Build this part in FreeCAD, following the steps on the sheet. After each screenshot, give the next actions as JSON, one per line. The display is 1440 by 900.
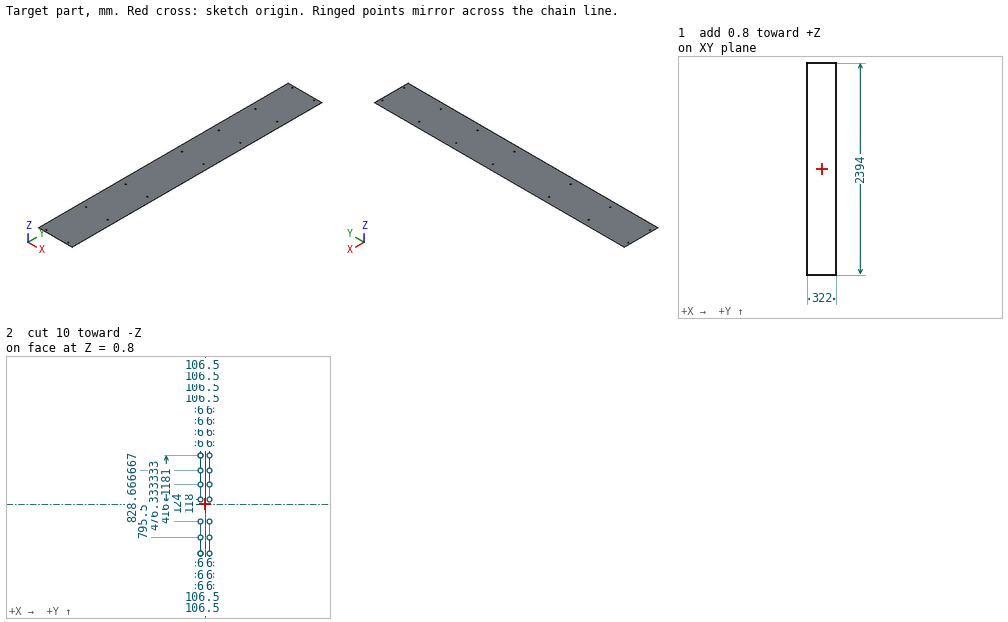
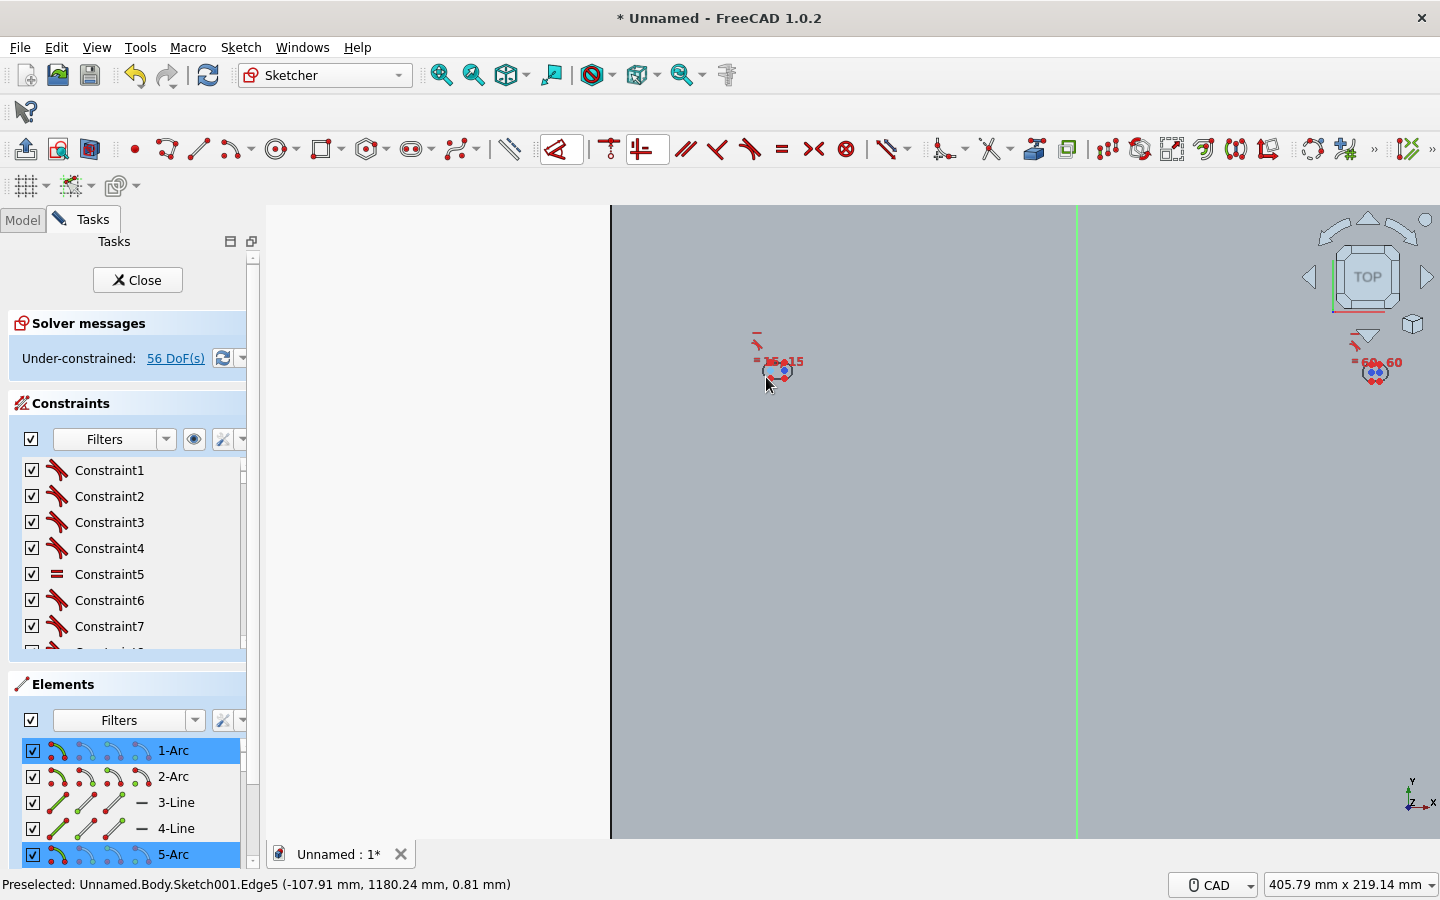
{"action": "left_click", "coordinate": [763, 371]}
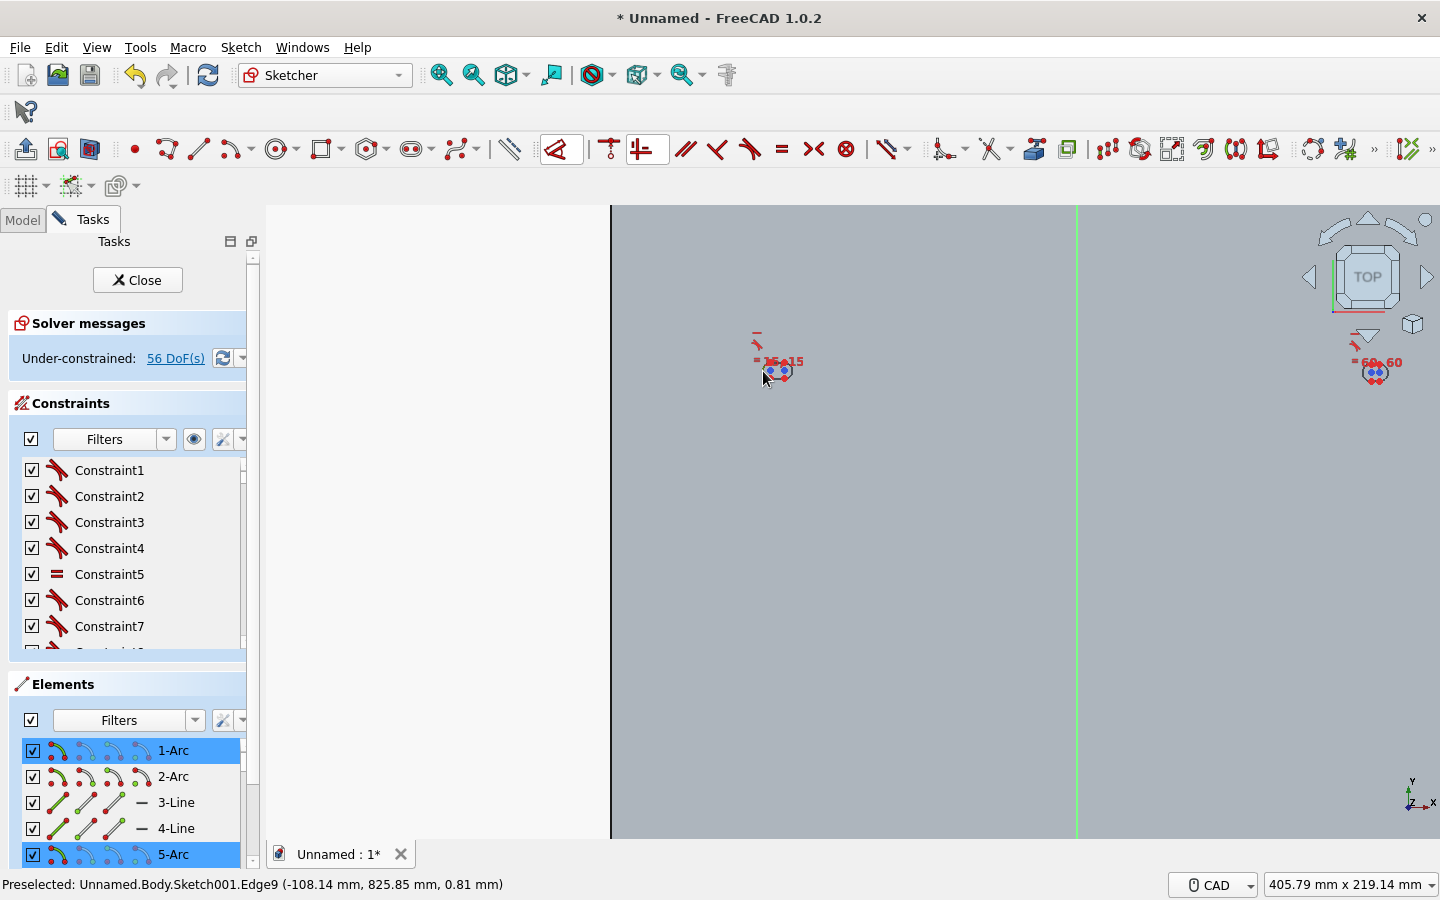
{"action": "scroll", "coordinate": [766, 377], "scroll_direction": "down", "scroll_amount": 14}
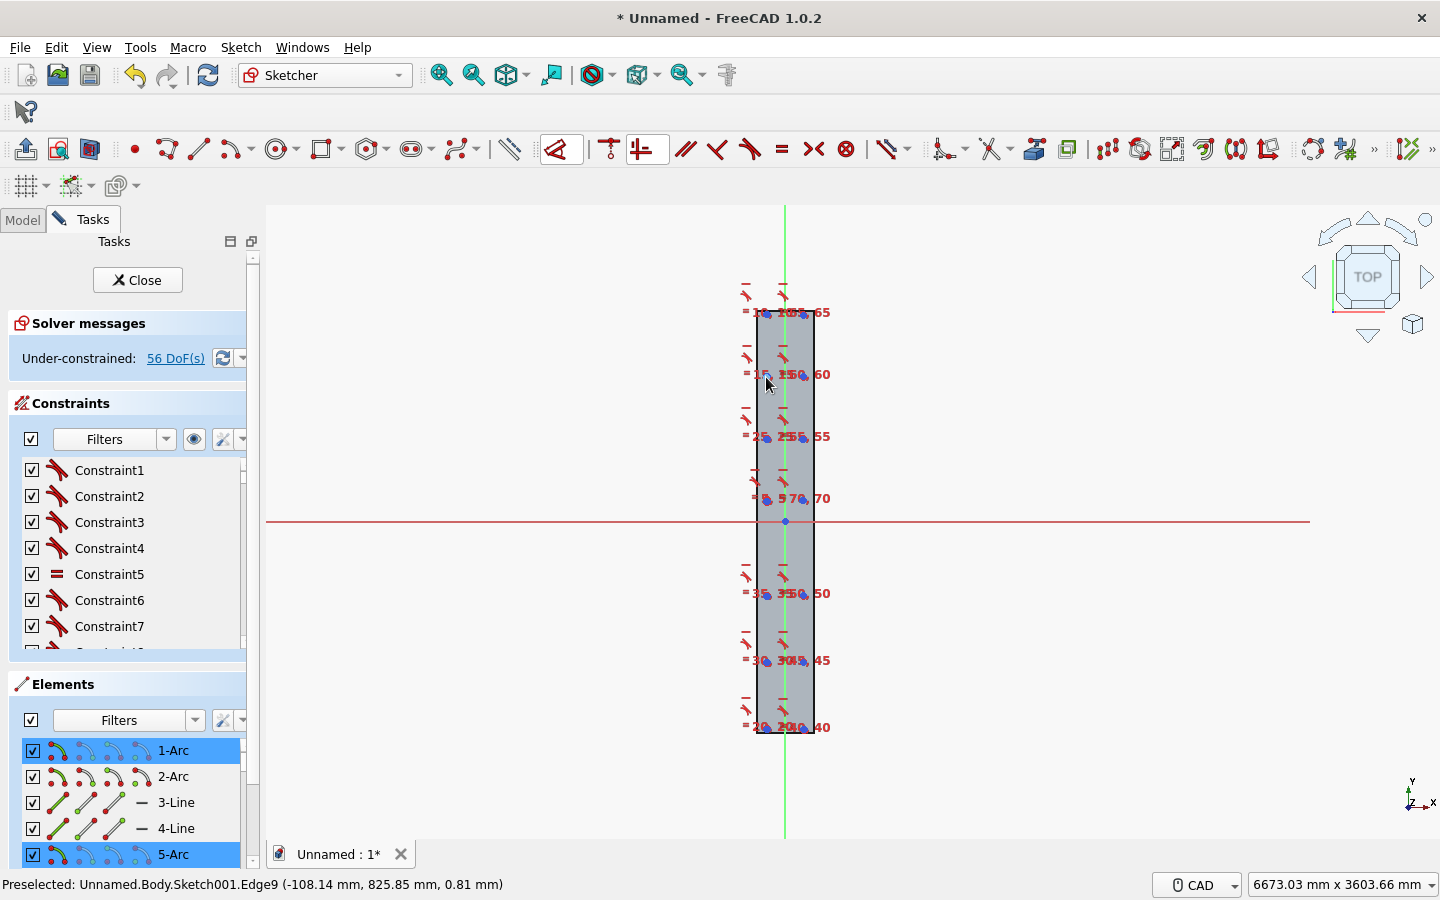
{"action": "scroll", "coordinate": [766, 729], "scroll_direction": "up", "scroll_amount": 14}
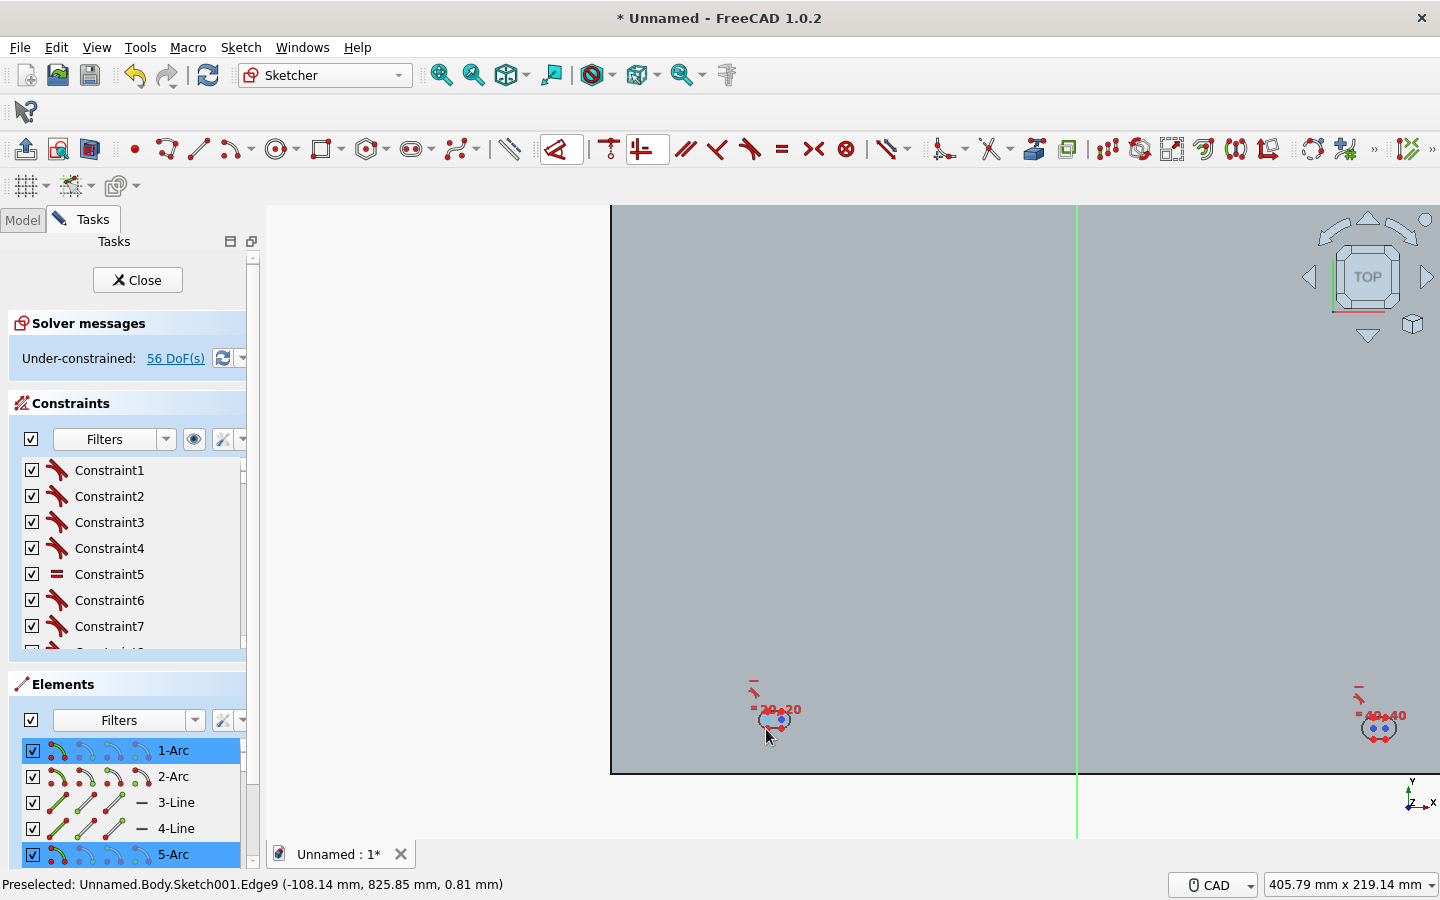
{"action": "left_click", "coordinate": [759, 720]}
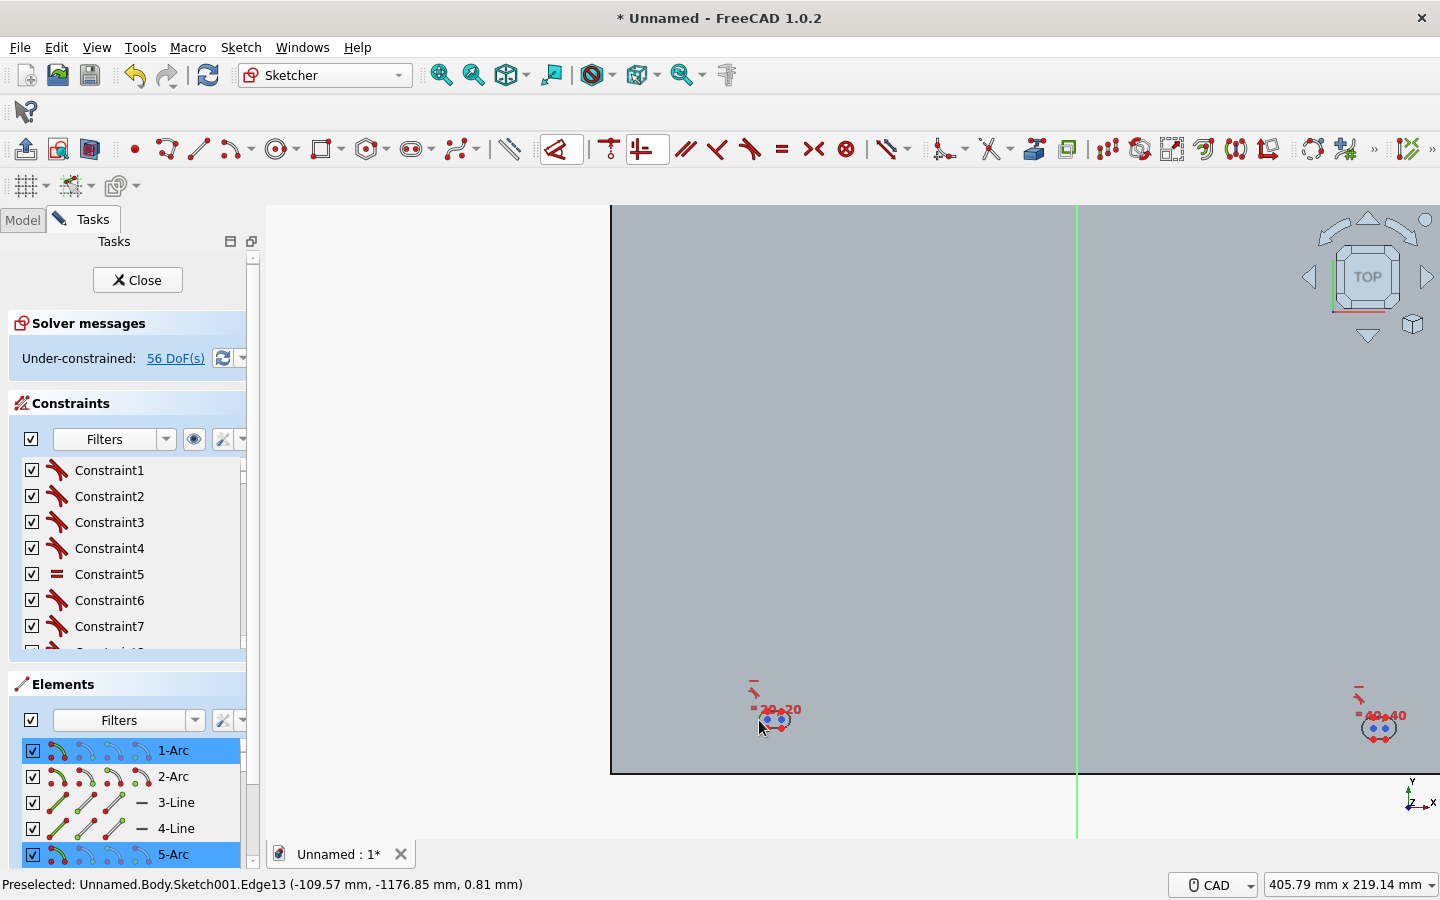
{"action": "scroll", "coordinate": [766, 730], "scroll_direction": "down", "scroll_amount": 14}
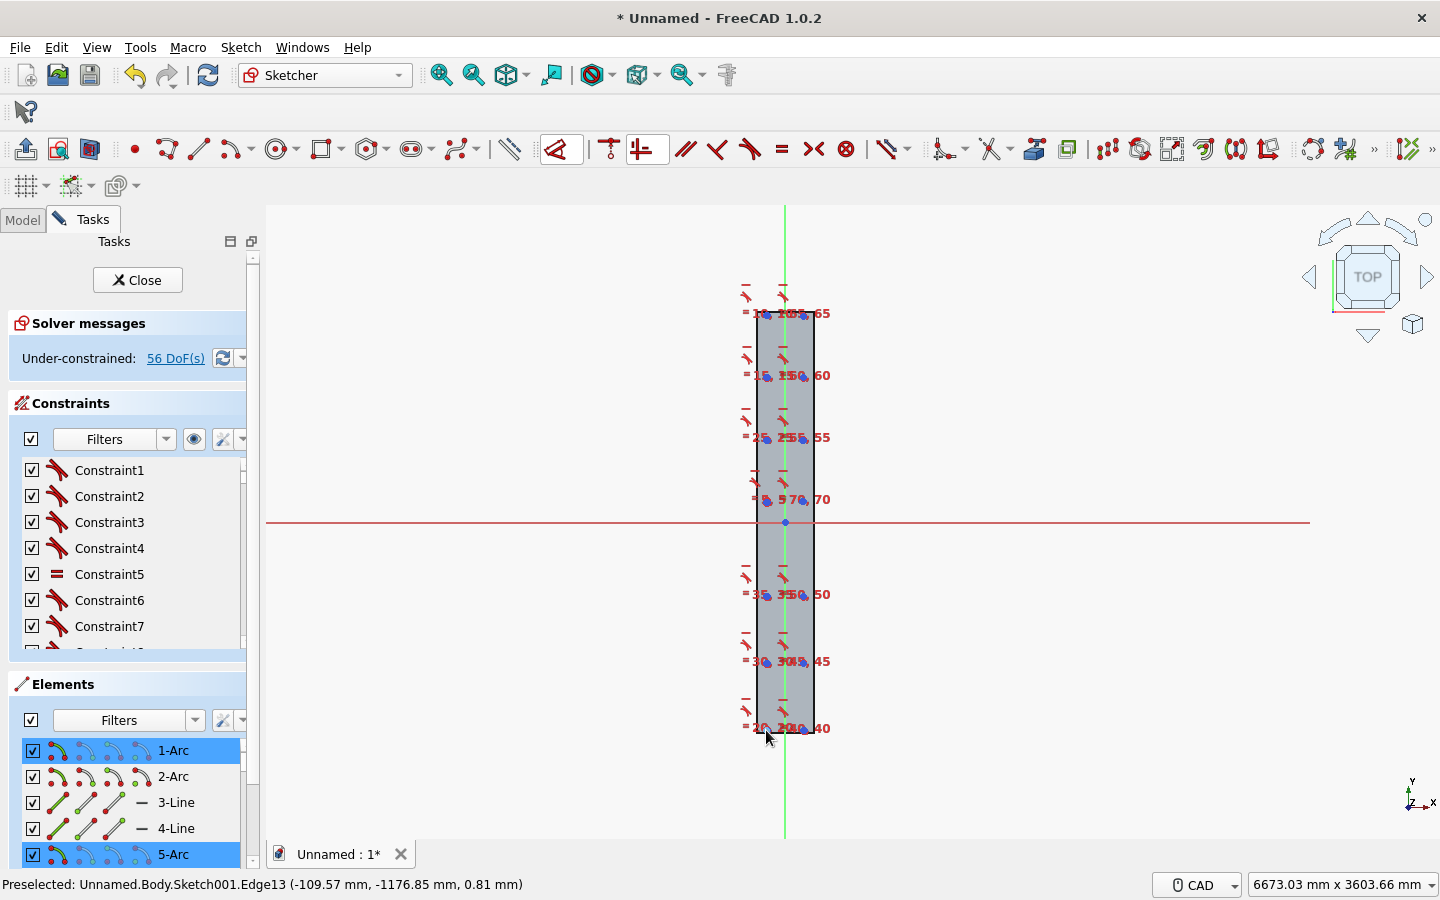
{"action": "scroll", "coordinate": [766, 440], "scroll_direction": "up", "scroll_amount": 14}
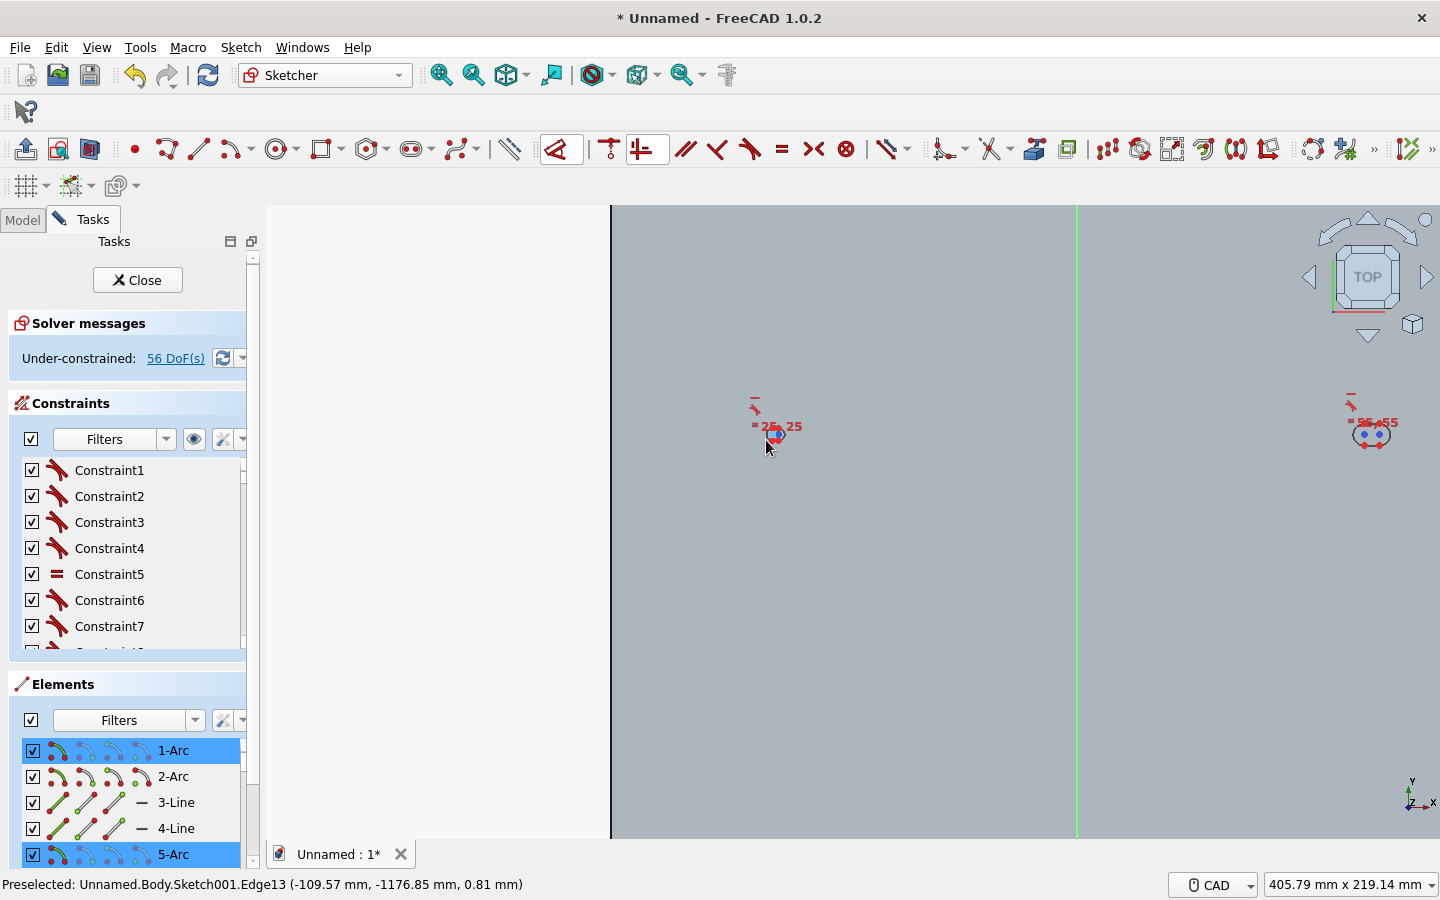
{"action": "left_click", "coordinate": [767, 434]}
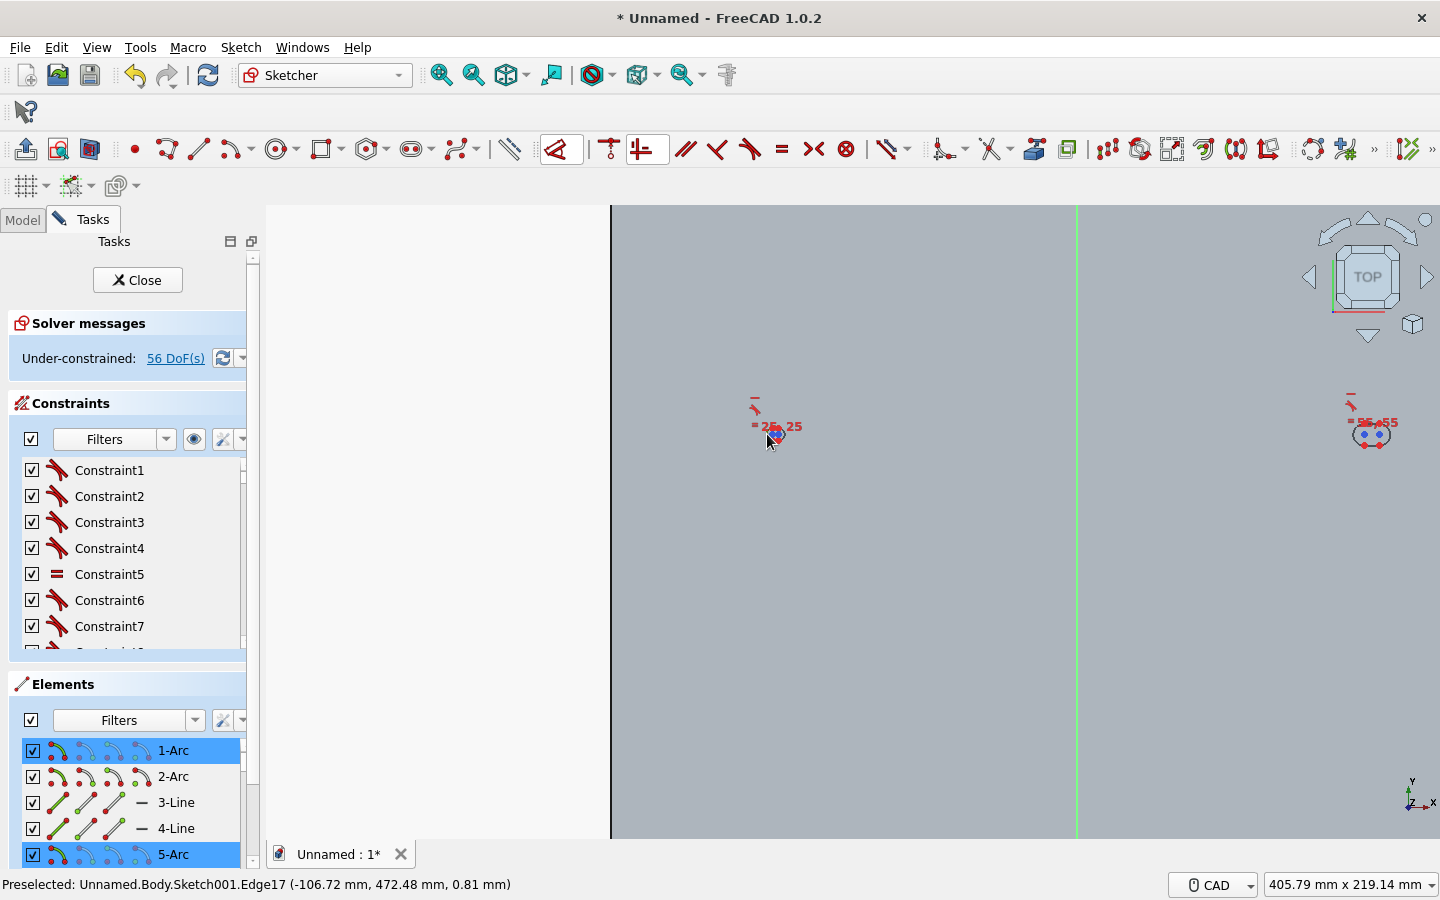
{"action": "scroll", "coordinate": [766, 439], "scroll_direction": "down", "scroll_amount": 14}